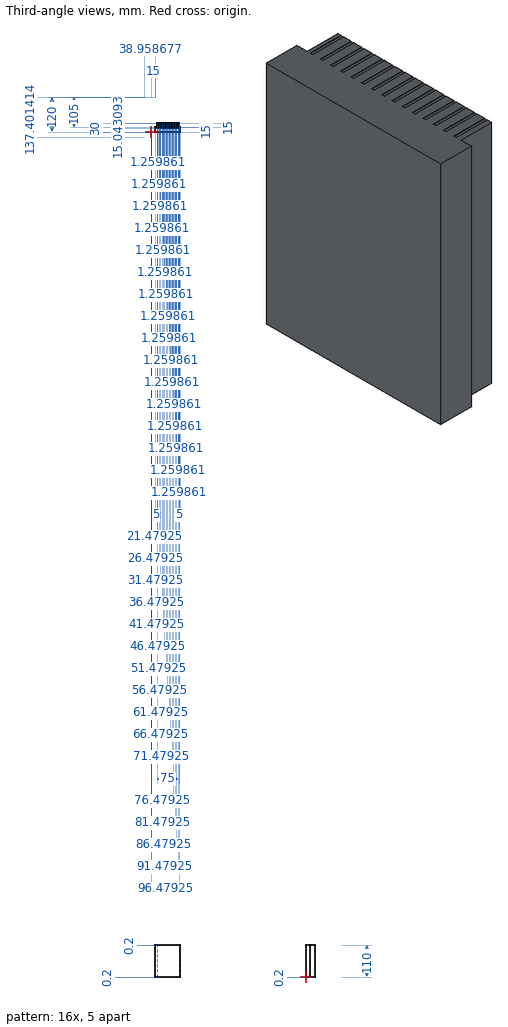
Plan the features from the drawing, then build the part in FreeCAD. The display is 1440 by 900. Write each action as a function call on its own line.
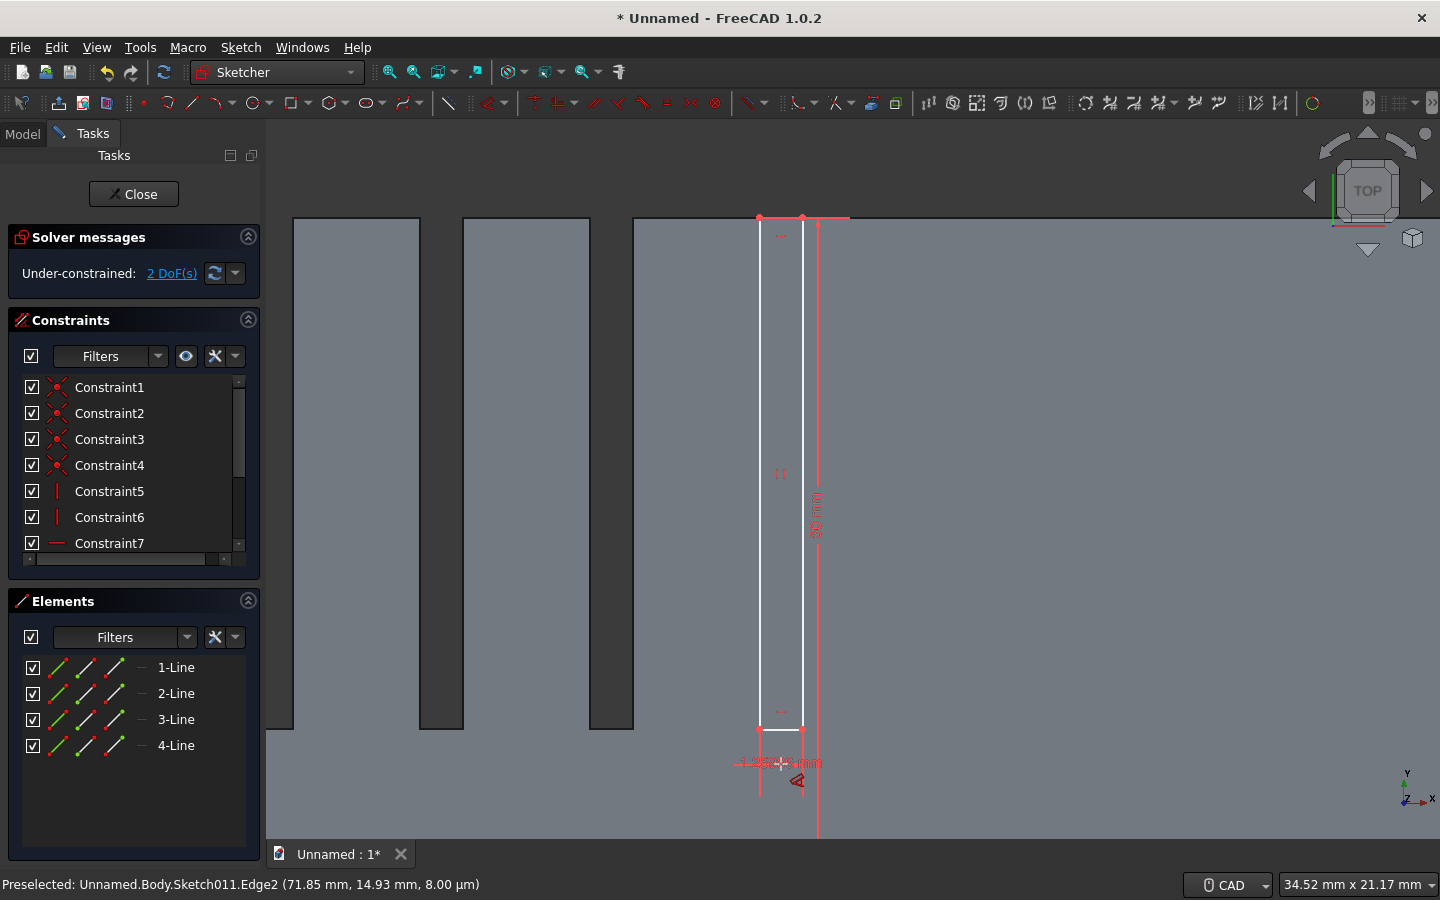
click(760, 371)
click(726, 474)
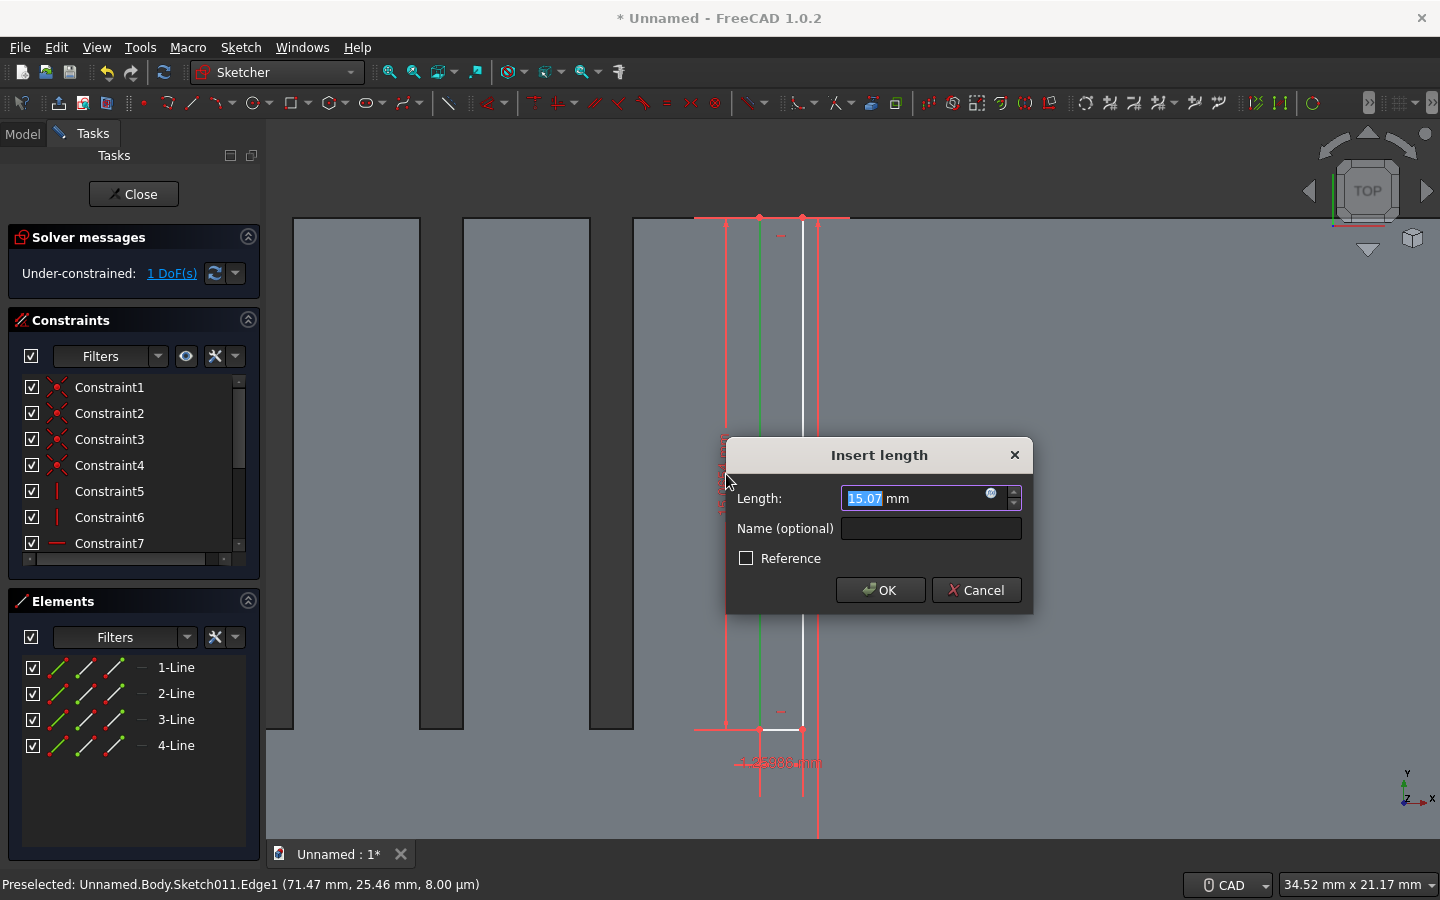
text(15.043093)
key(Return)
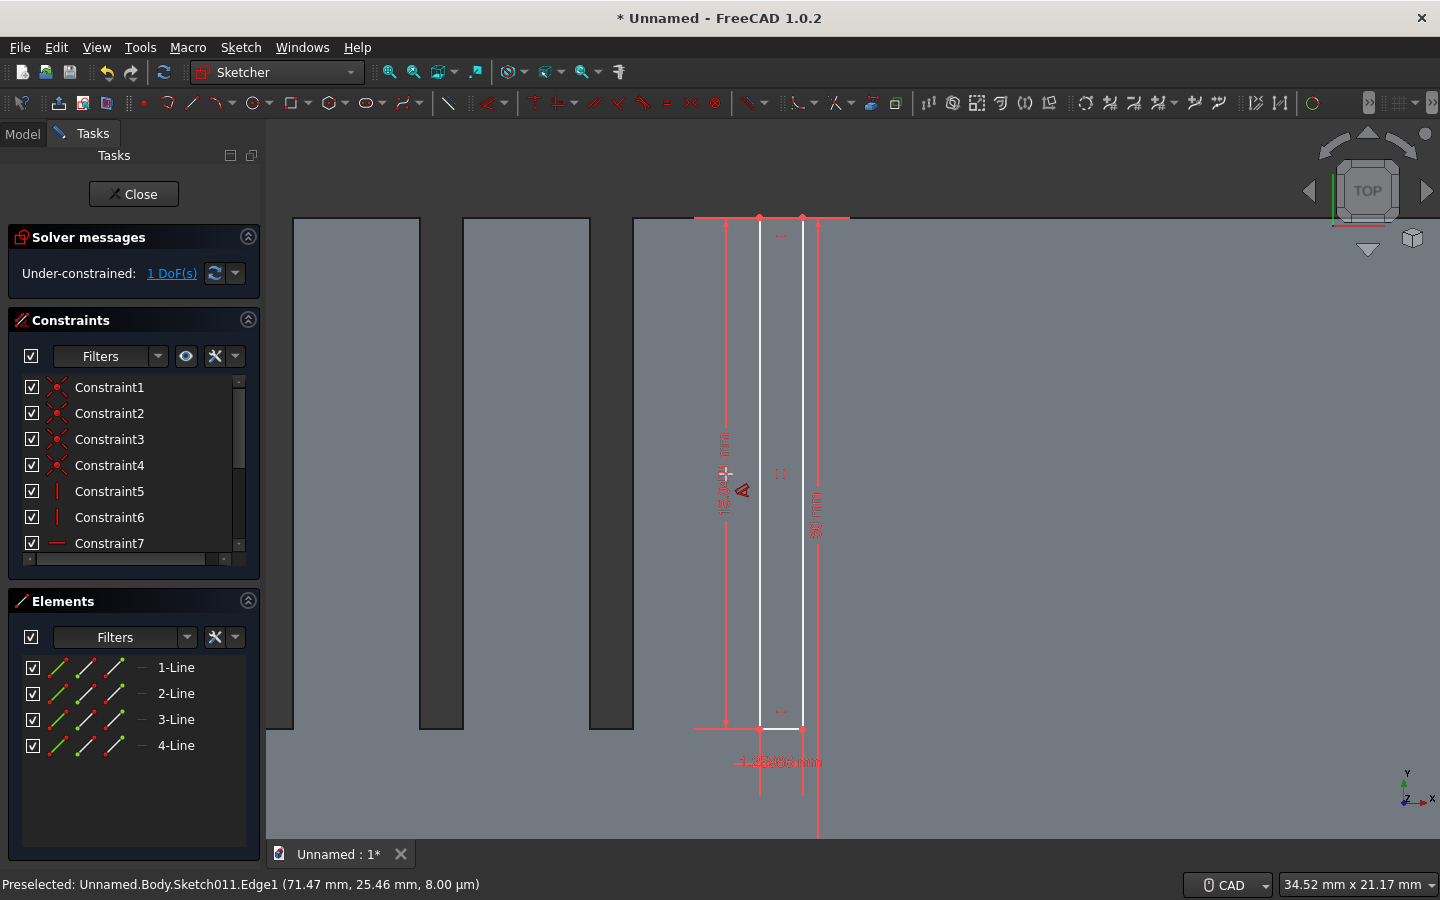
click(760, 218)
click(527, 184)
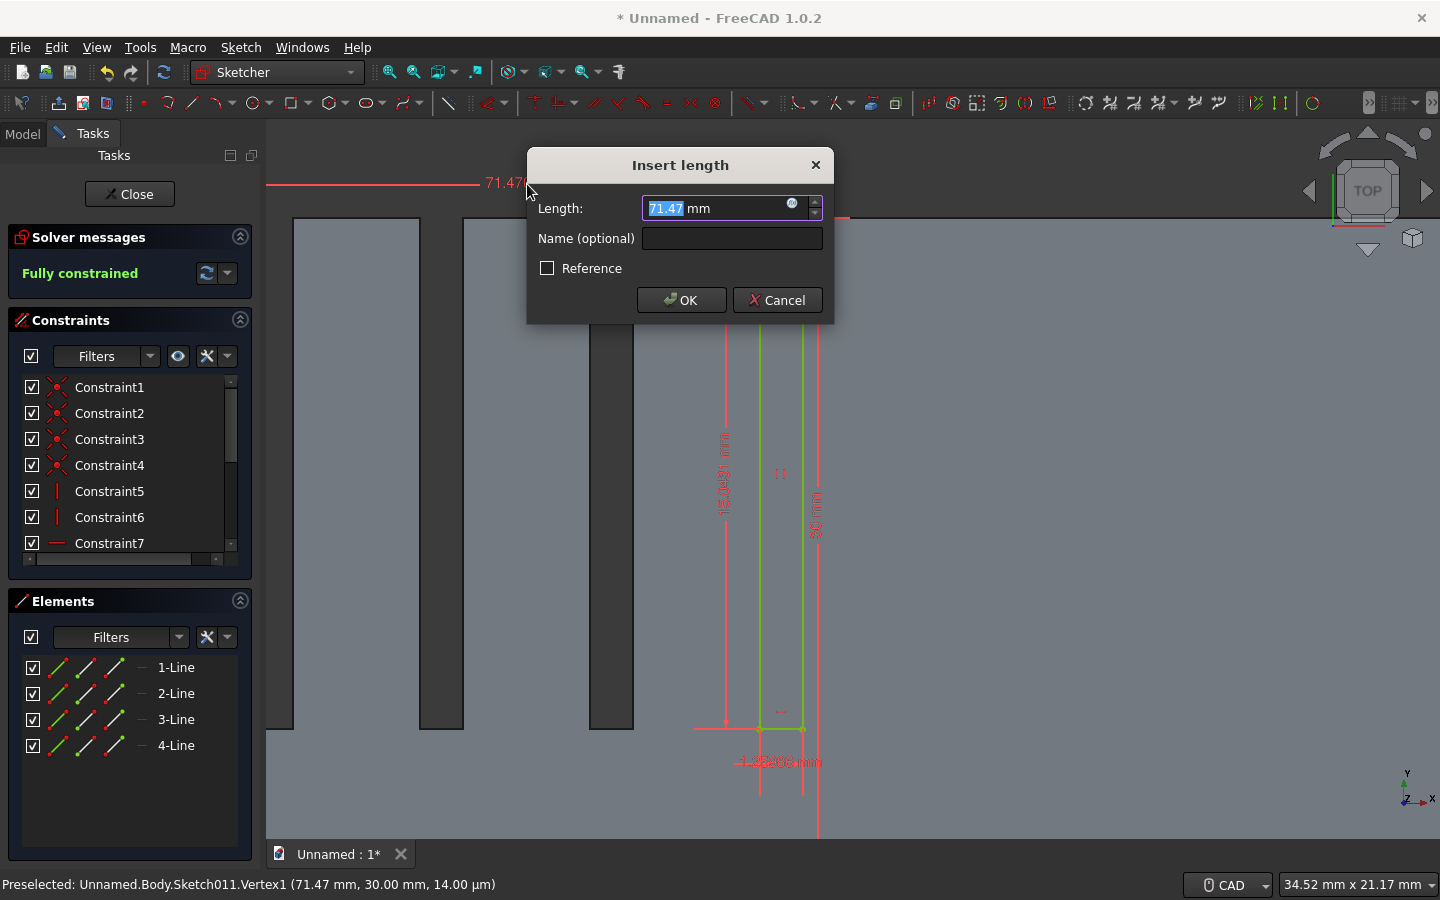
text(71.47925)
key(Return)
key(Escape)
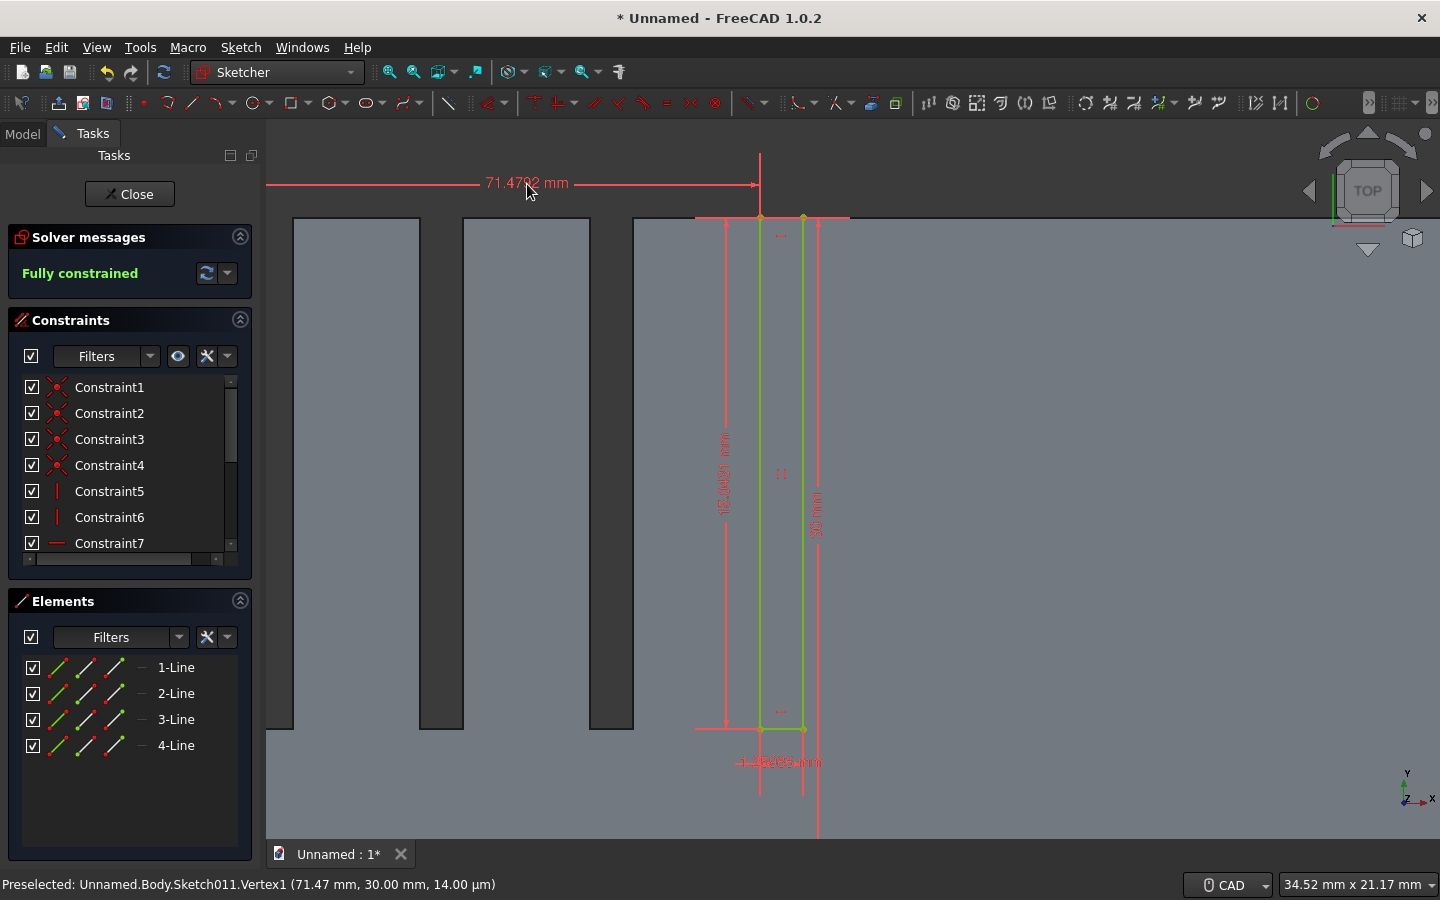
click(130, 194)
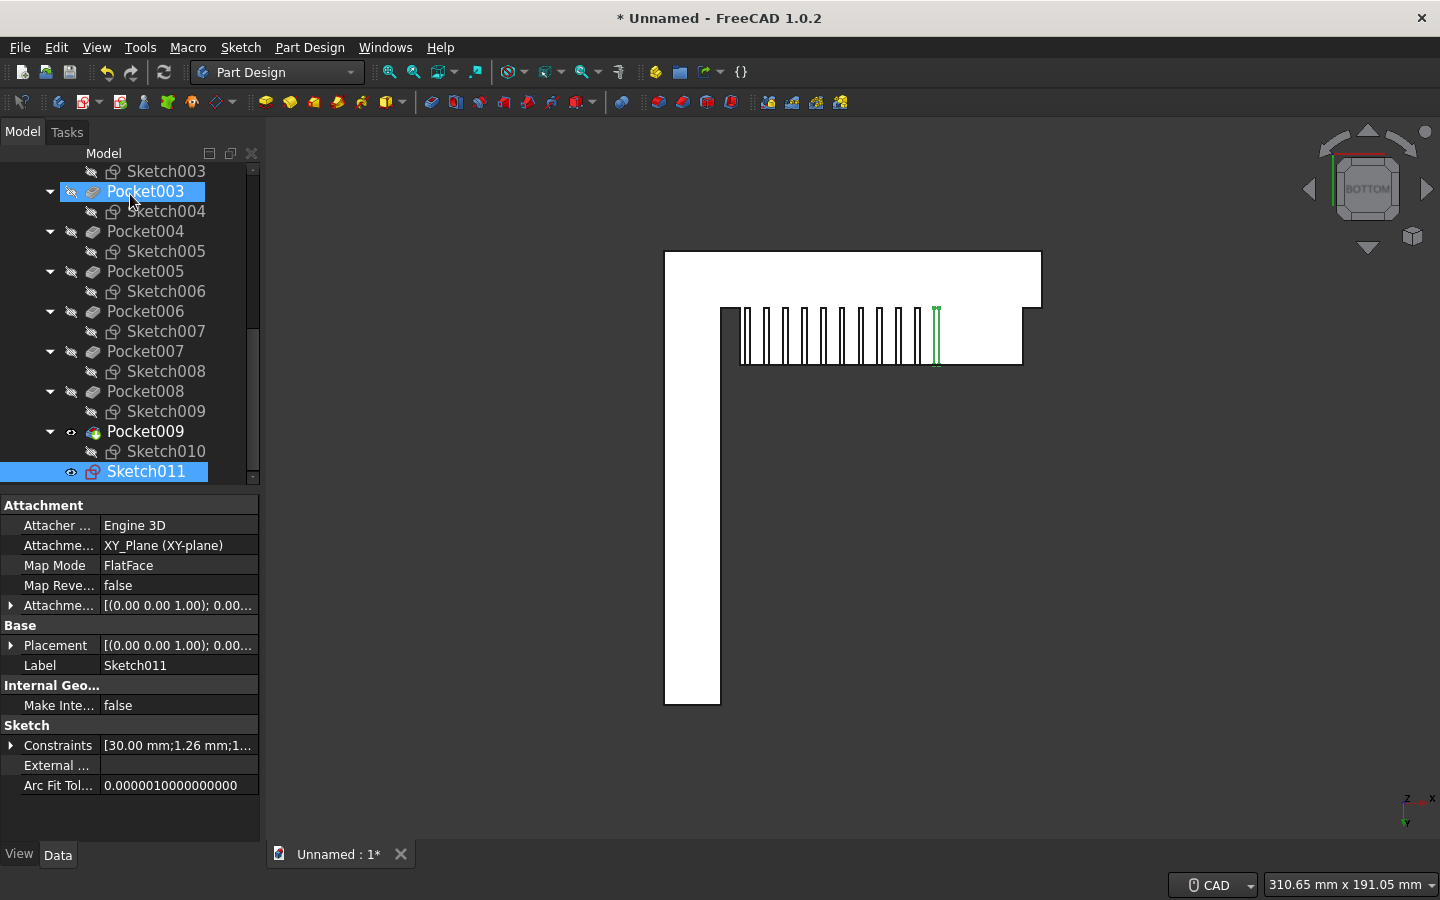
click(432, 102)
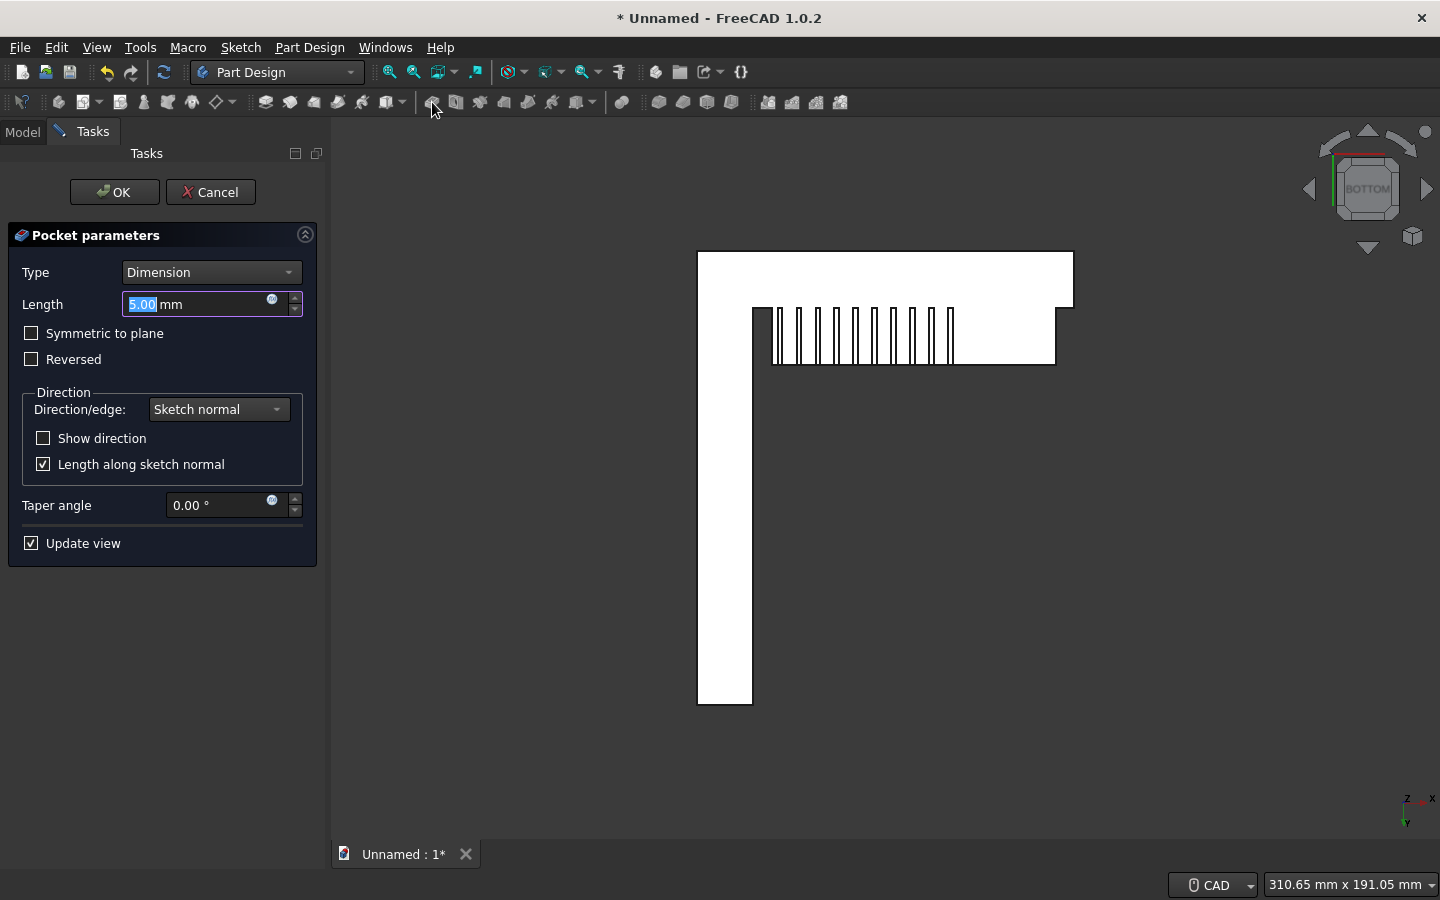
text(0.2)
key(Tab)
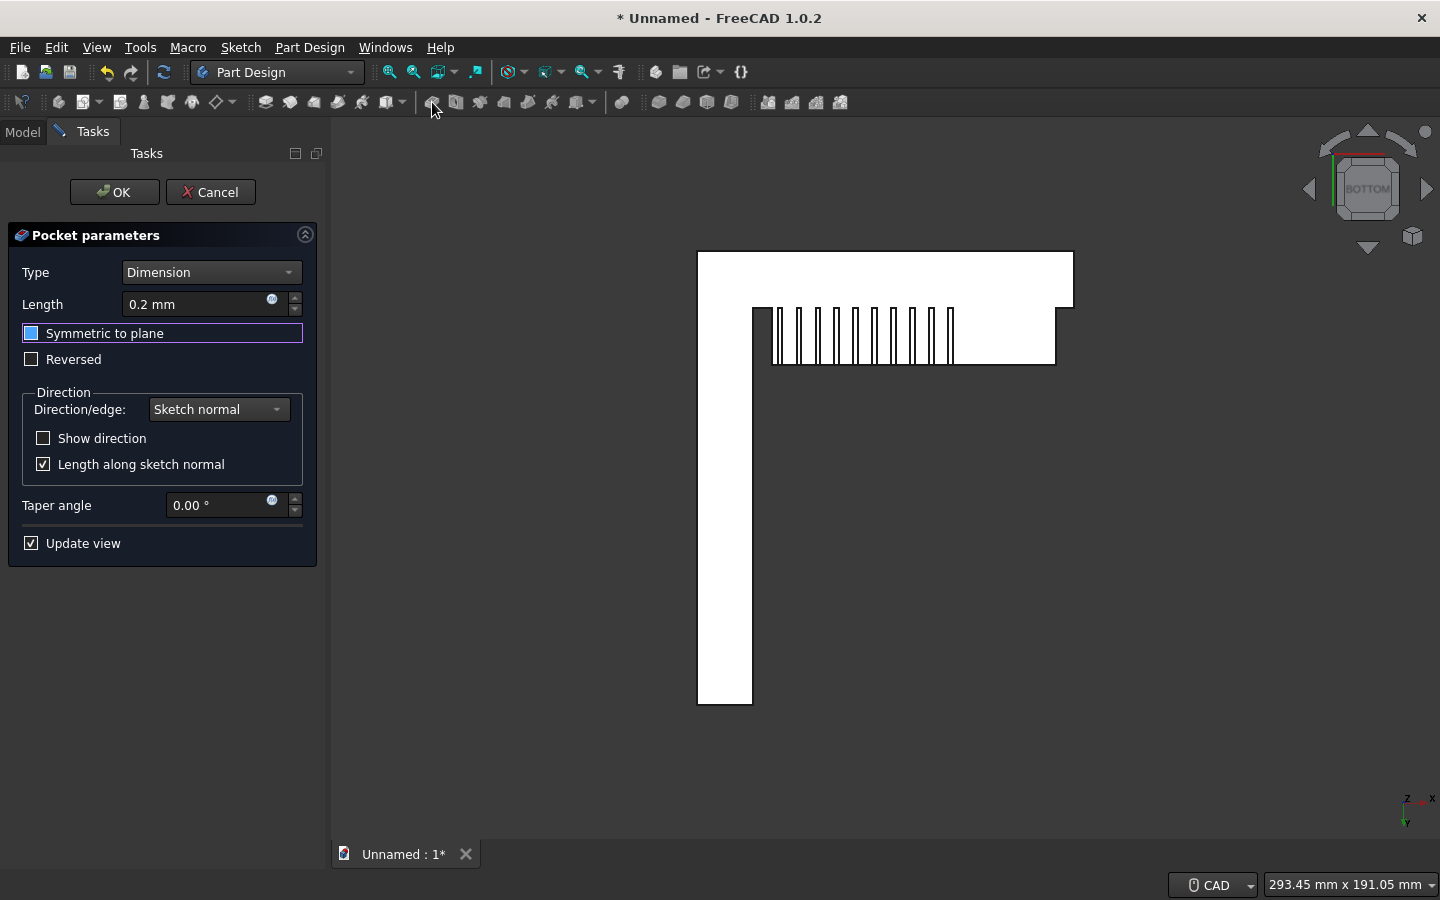
click(30, 359)